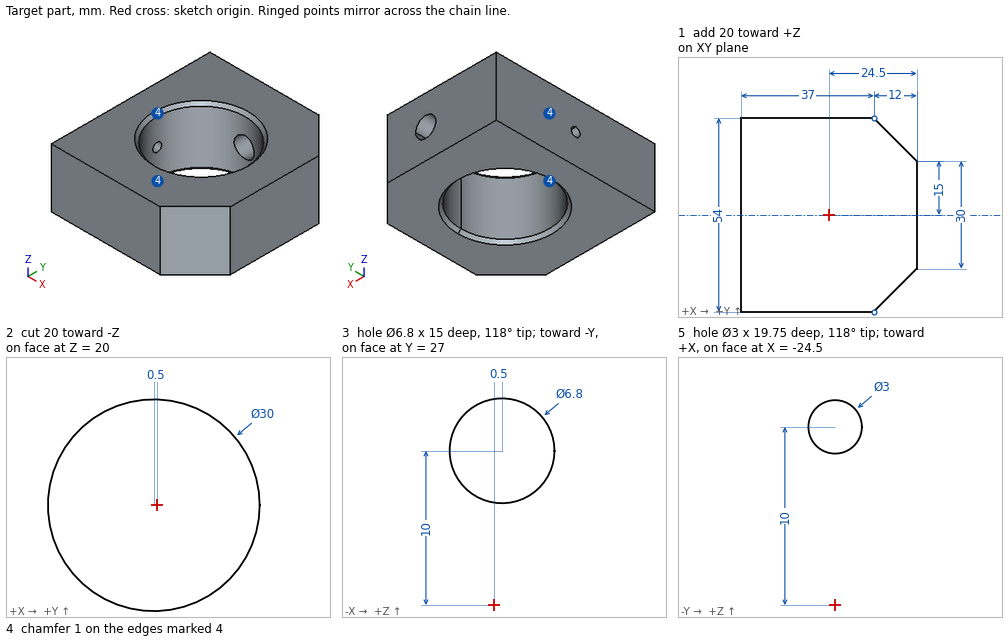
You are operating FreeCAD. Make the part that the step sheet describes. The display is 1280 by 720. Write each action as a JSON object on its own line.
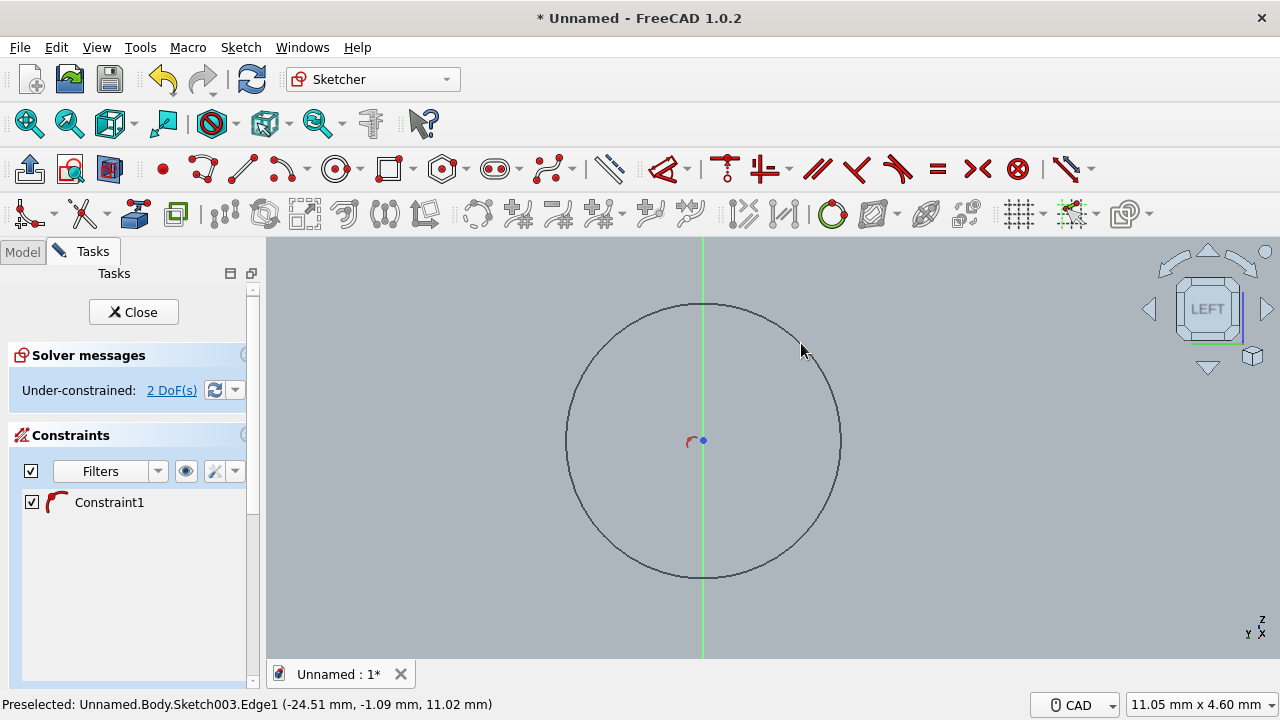
{"action": "left_click", "coordinate": [664, 170]}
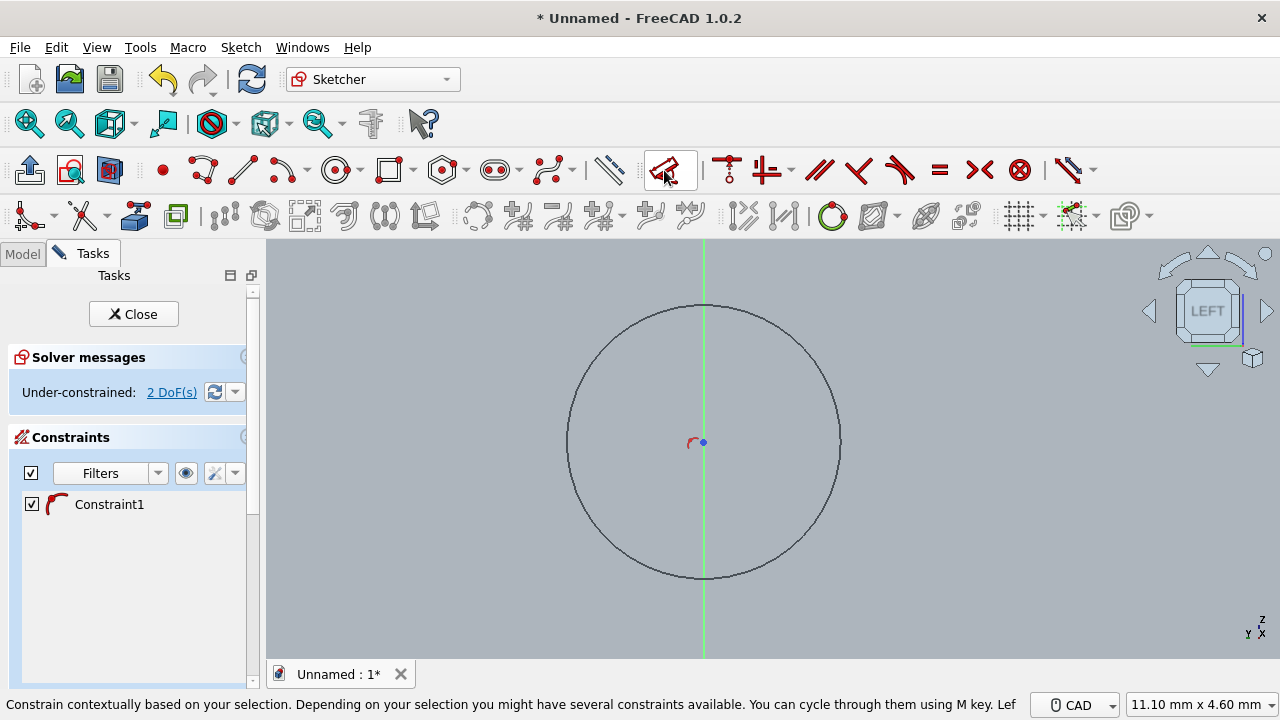
{"action": "left_click", "coordinate": [800, 345]}
{"action": "left_click", "coordinate": [823, 322]}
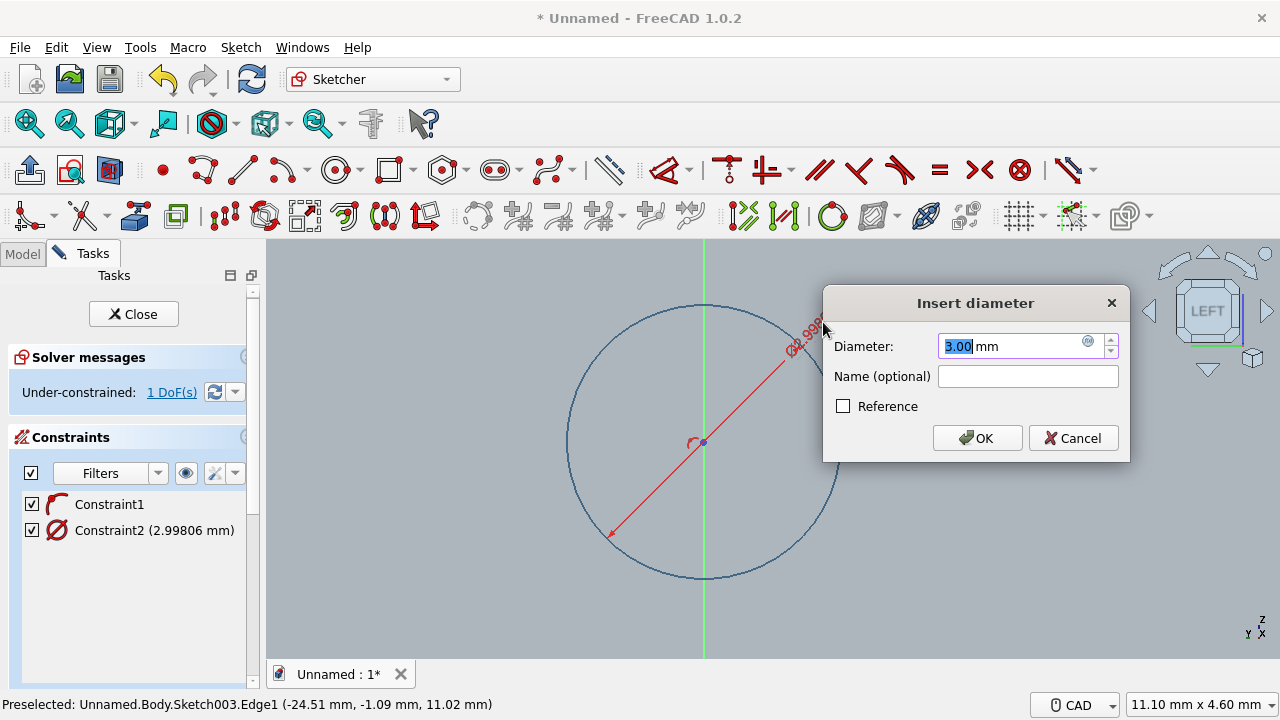
{"action": "type", "text": "3"}
{"action": "key", "text": "Return"}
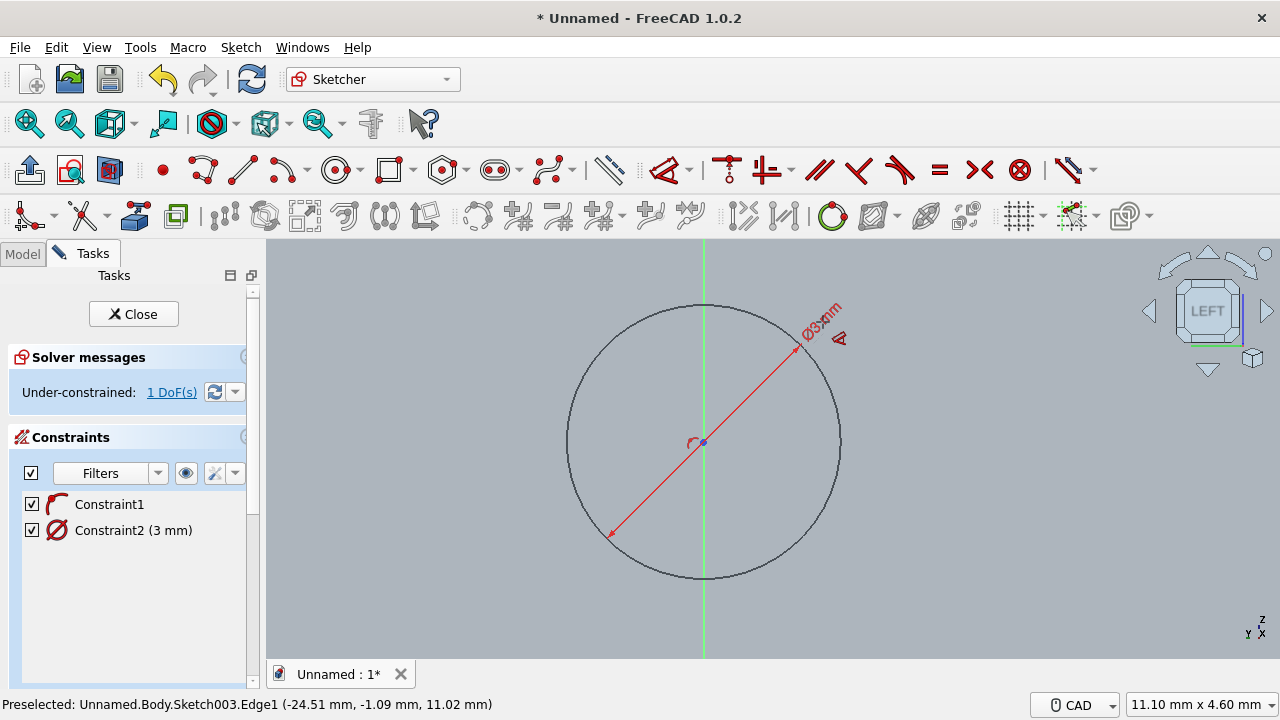
{"action": "left_click", "coordinate": [704, 442]}
{"action": "left_click", "coordinate": [738, 537]}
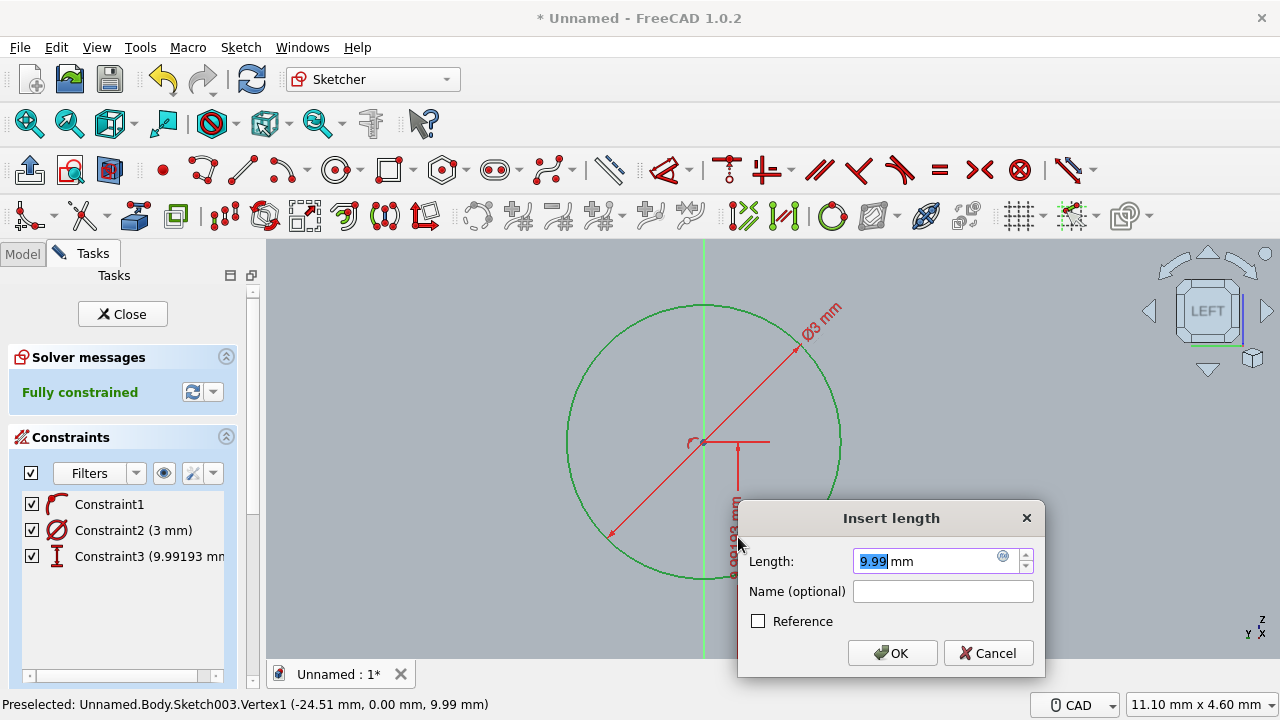
{"action": "type", "text": "10"}
{"action": "key", "text": "Return"}
{"action": "key", "text": "Escape"}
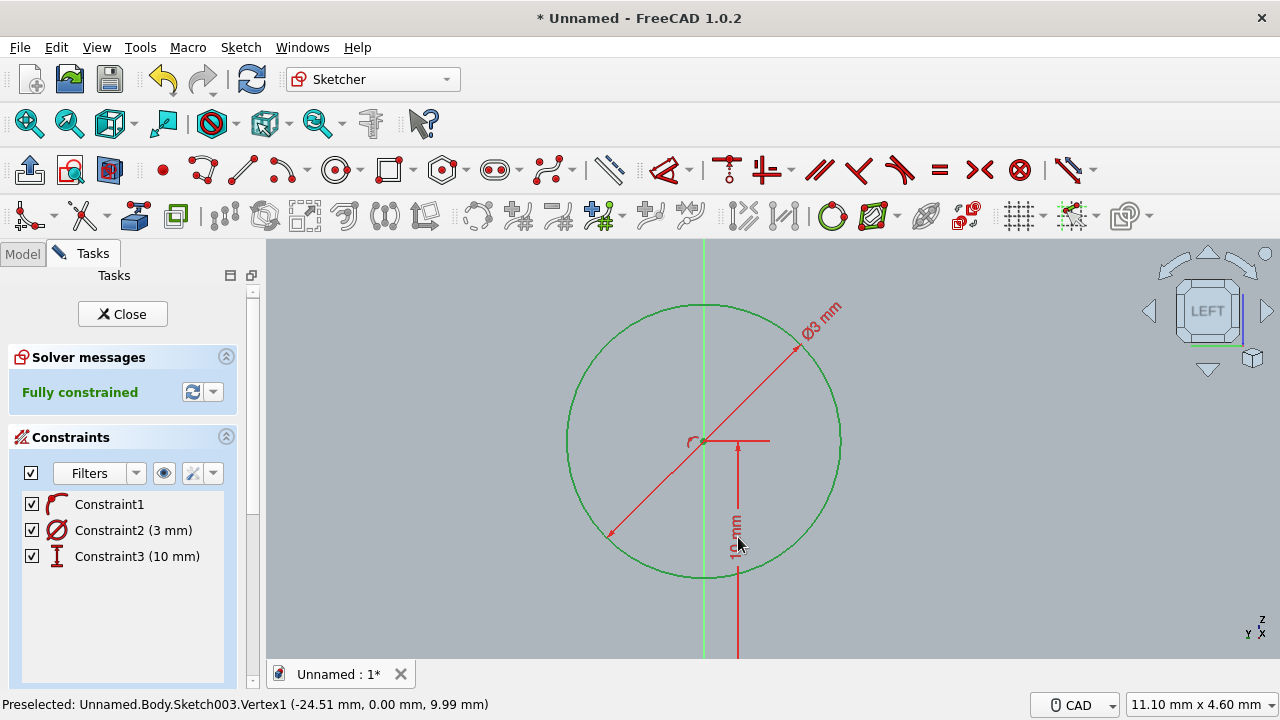
{"action": "left_click", "coordinate": [123, 314]}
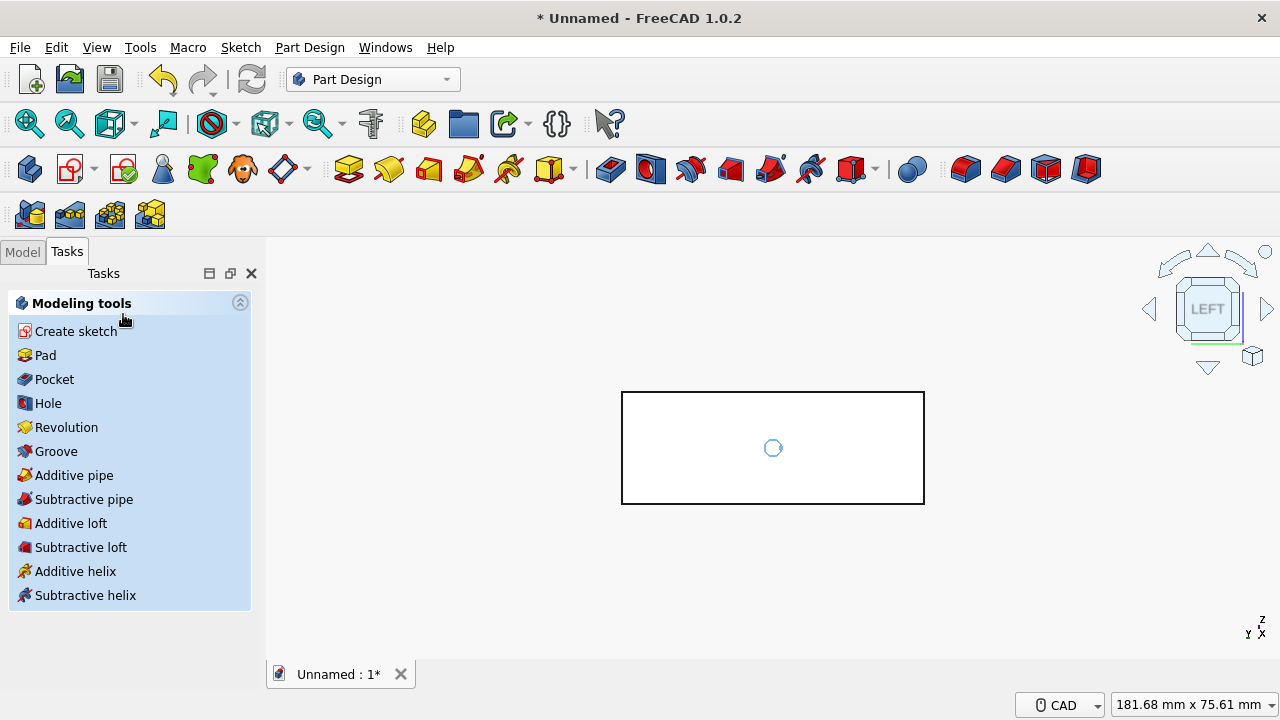
{"action": "left_click", "coordinate": [652, 170]}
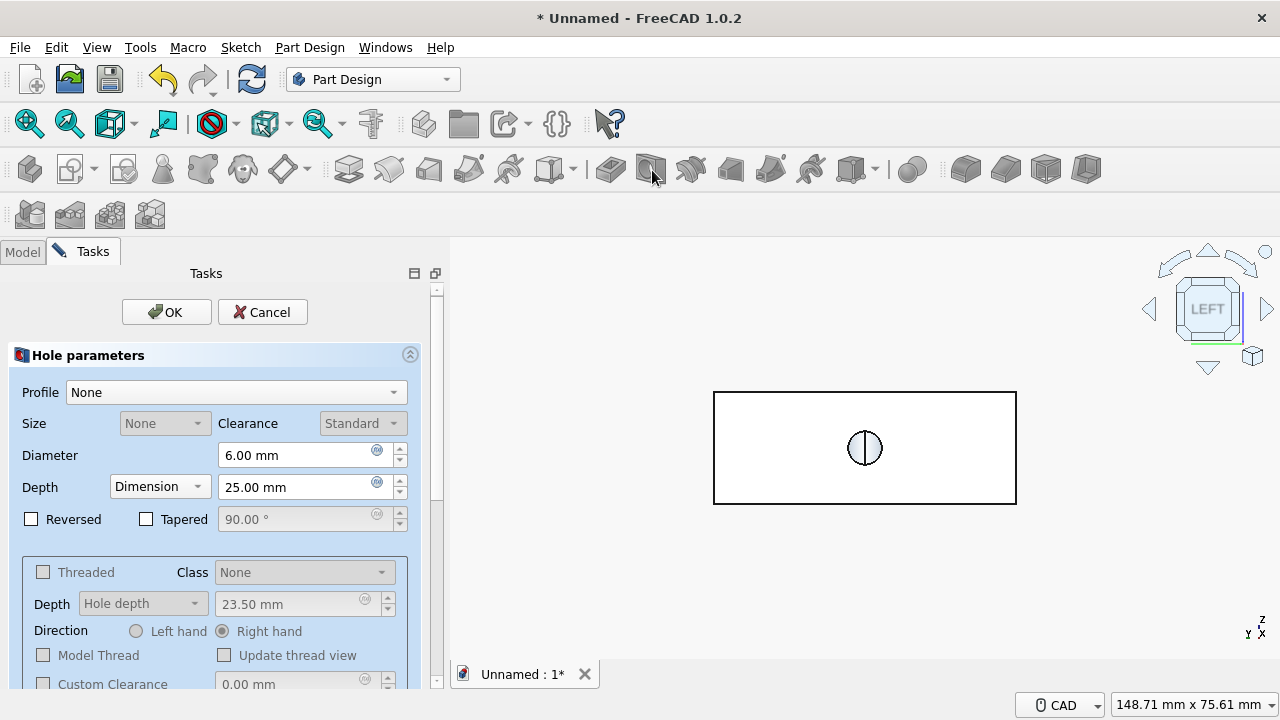
{"action": "triple_click", "coordinate": [305, 455]}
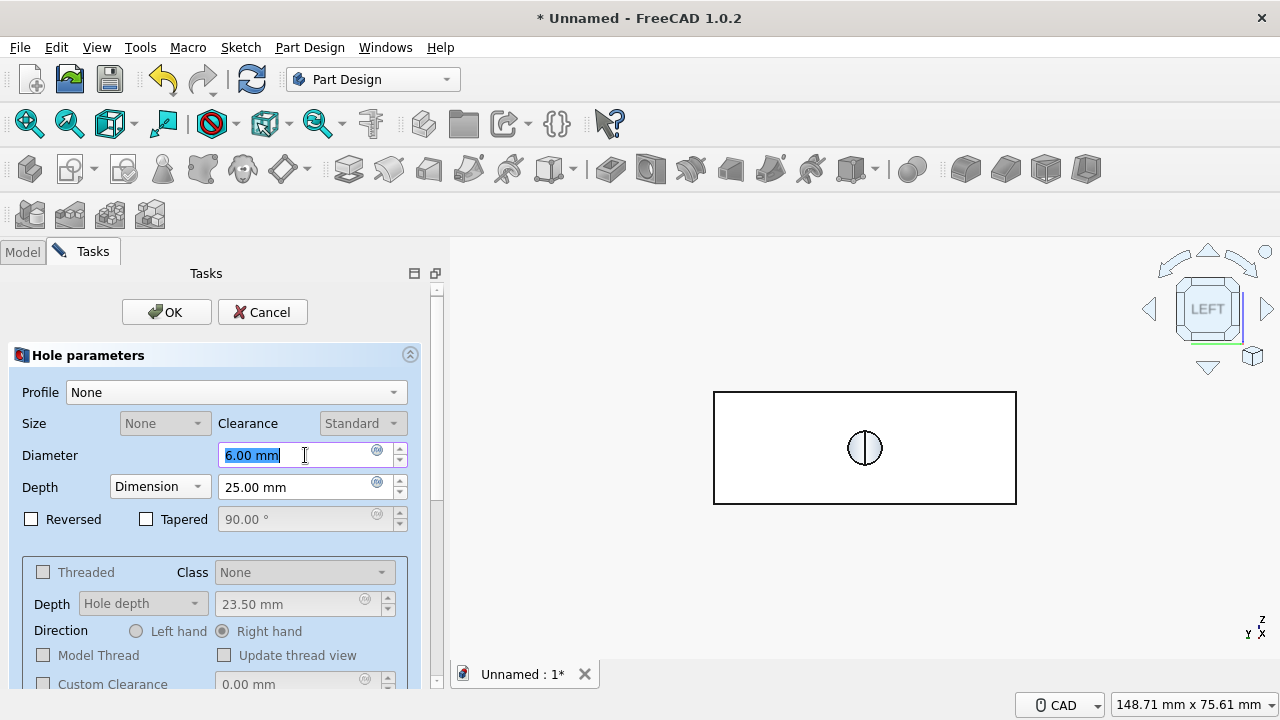
{"action": "type", "text": "3"}
{"action": "key", "text": "Tab"}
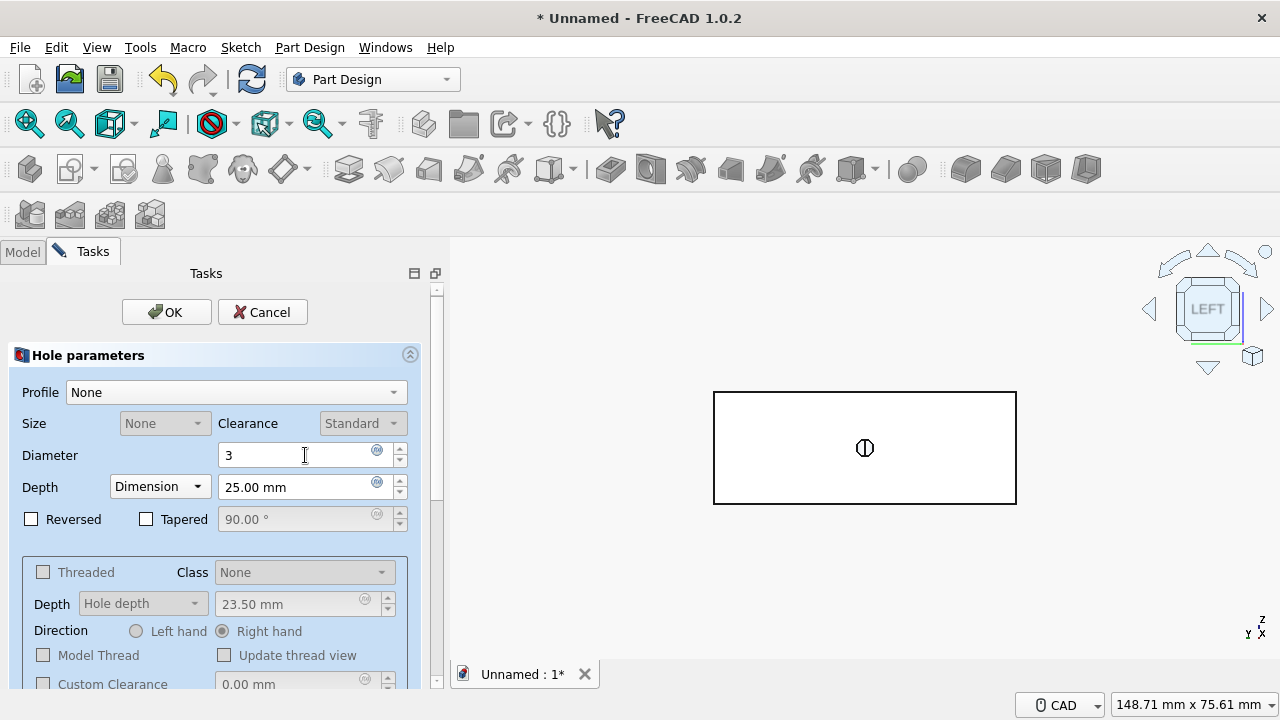
{"action": "triple_click", "coordinate": [305, 487]}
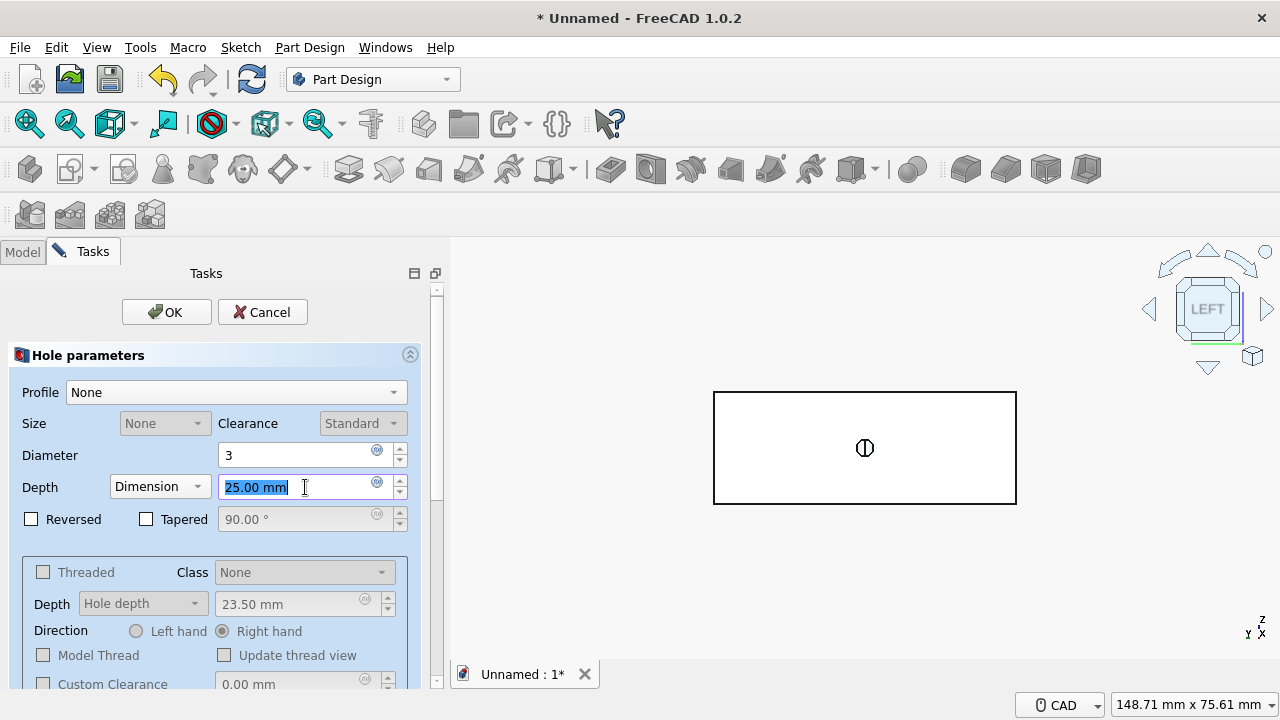
{"action": "type", "text": "19.75"}
{"action": "key", "text": "Tab"}